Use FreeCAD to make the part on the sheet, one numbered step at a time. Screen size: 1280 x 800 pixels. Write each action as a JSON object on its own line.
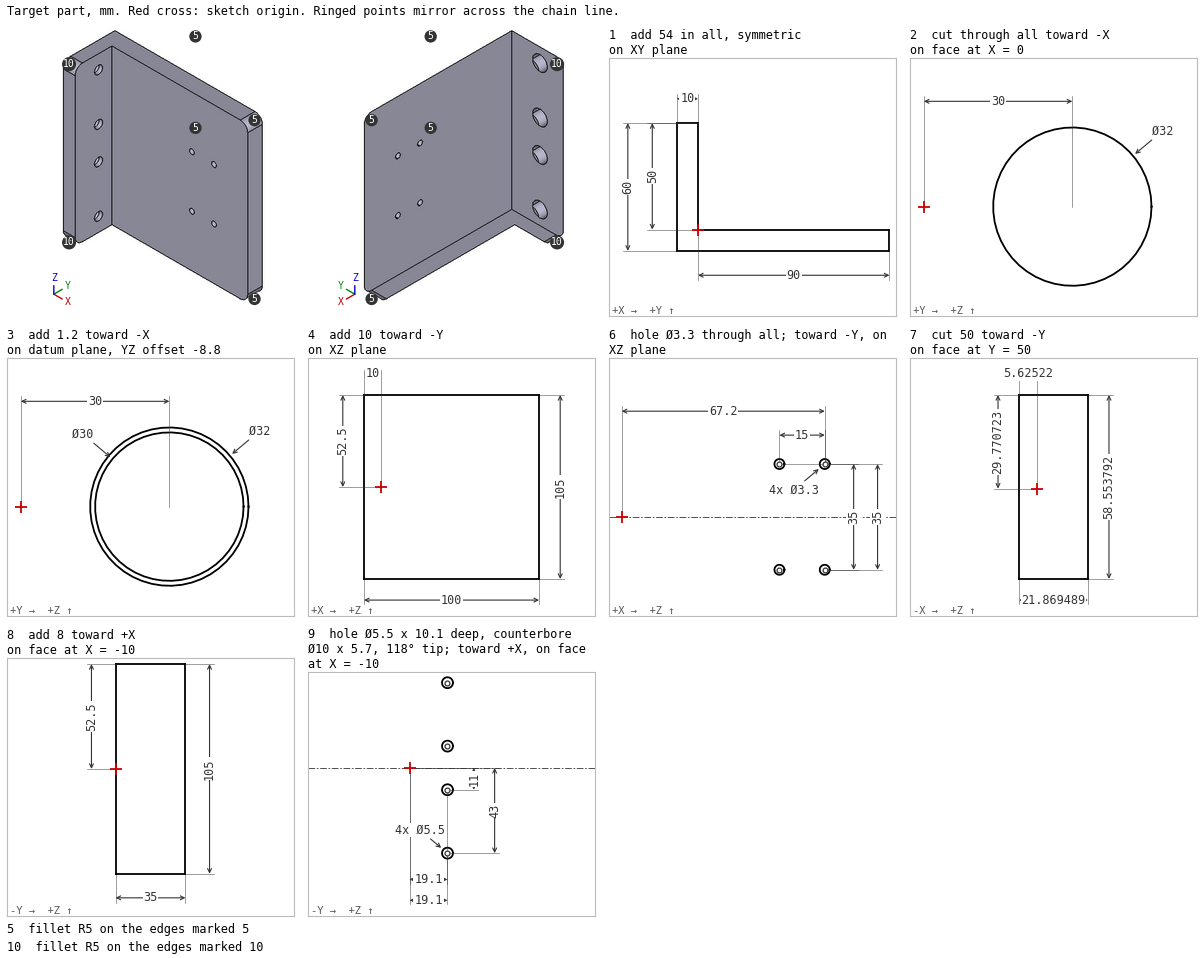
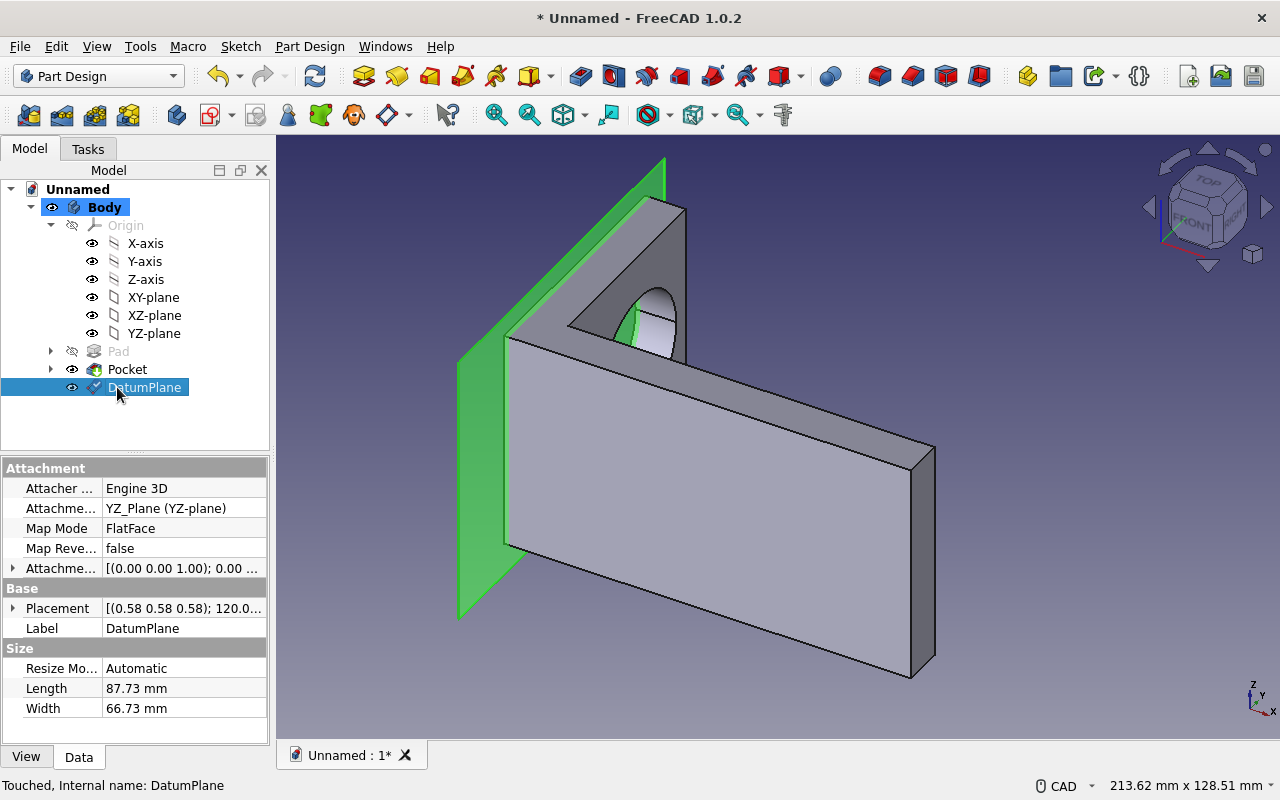
{"action": "left_click", "coordinate": [210, 116]}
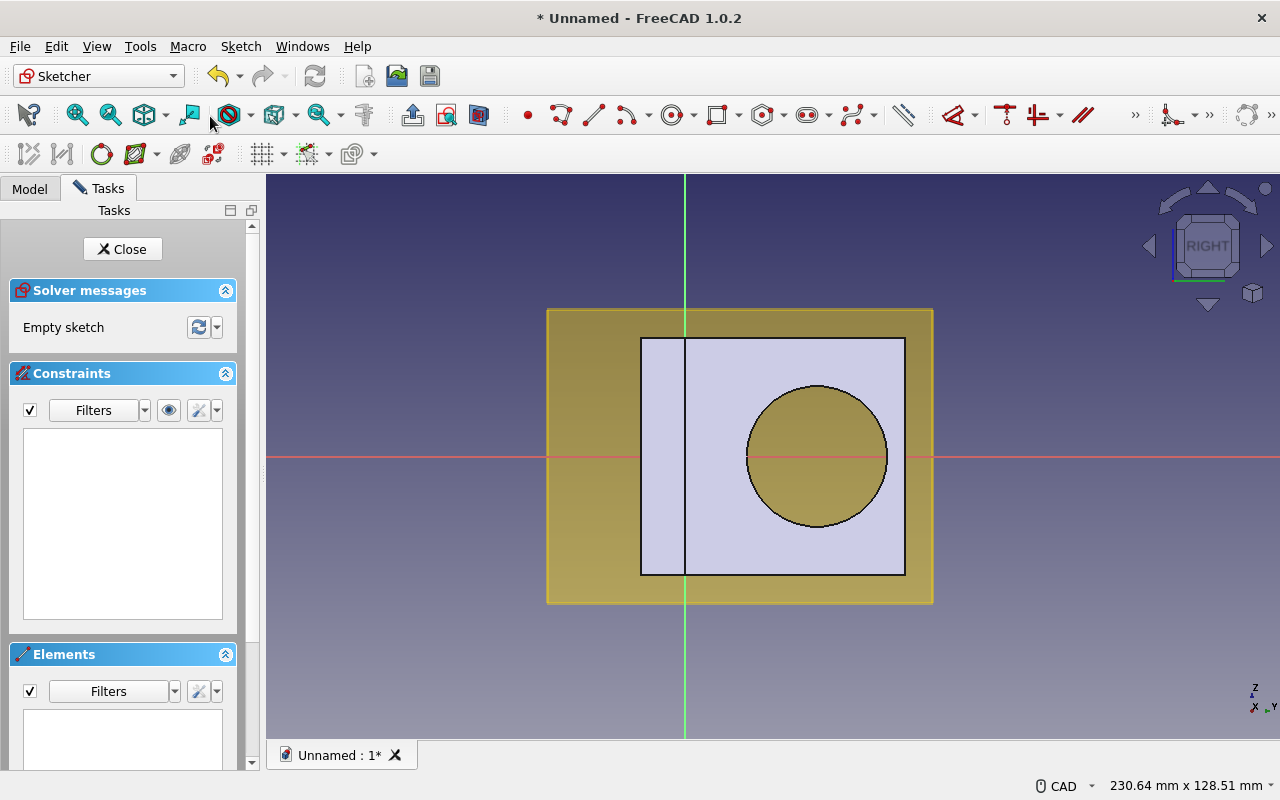
{"action": "left_click", "coordinate": [479, 116]}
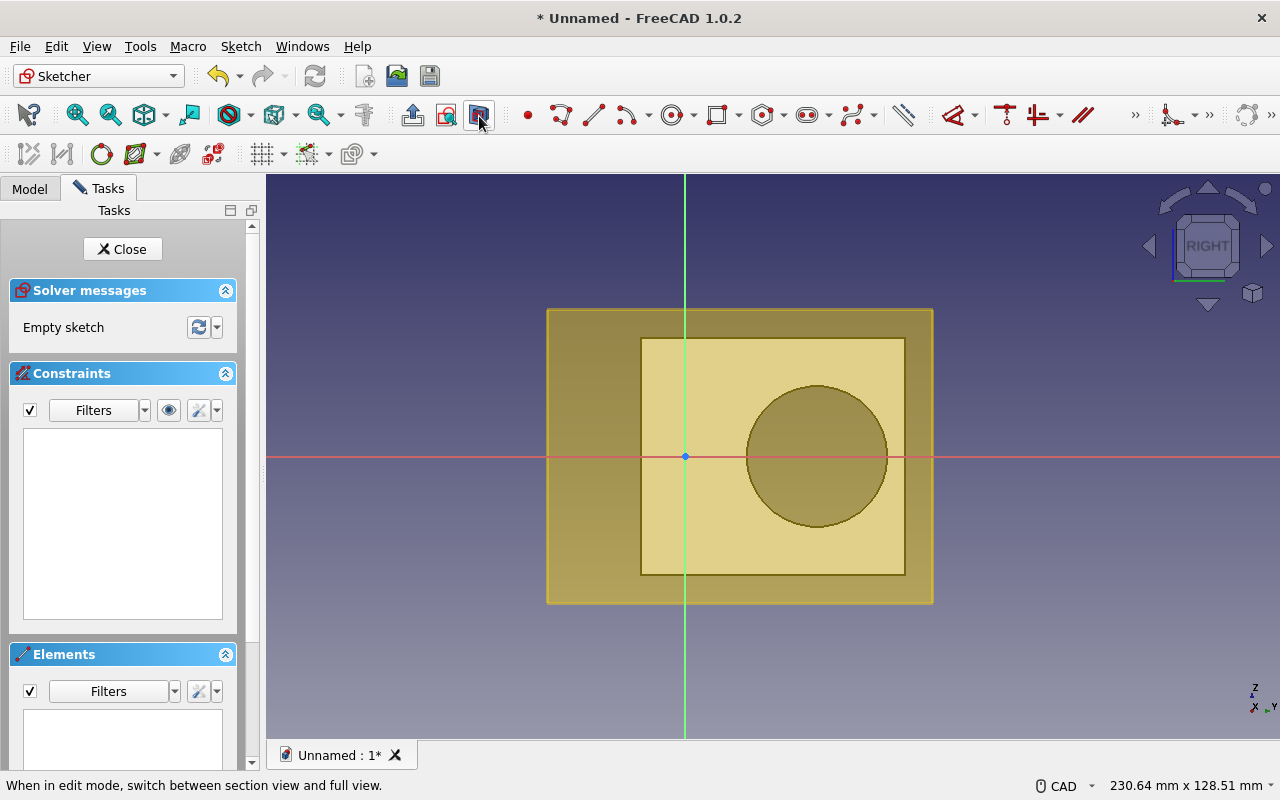
{"action": "scroll", "coordinate": [834, 456], "scroll_direction": "up", "scroll_amount": 5}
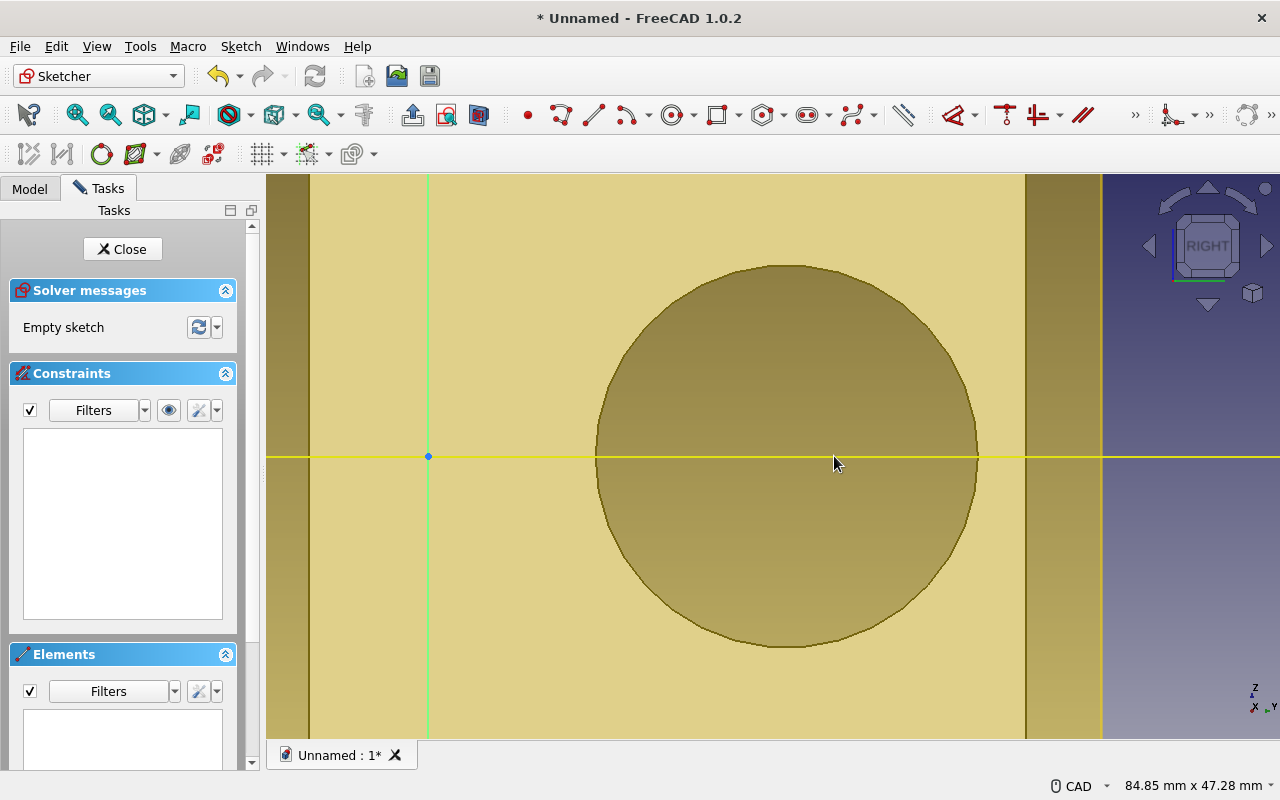
{"action": "left_click", "coordinate": [672, 116]}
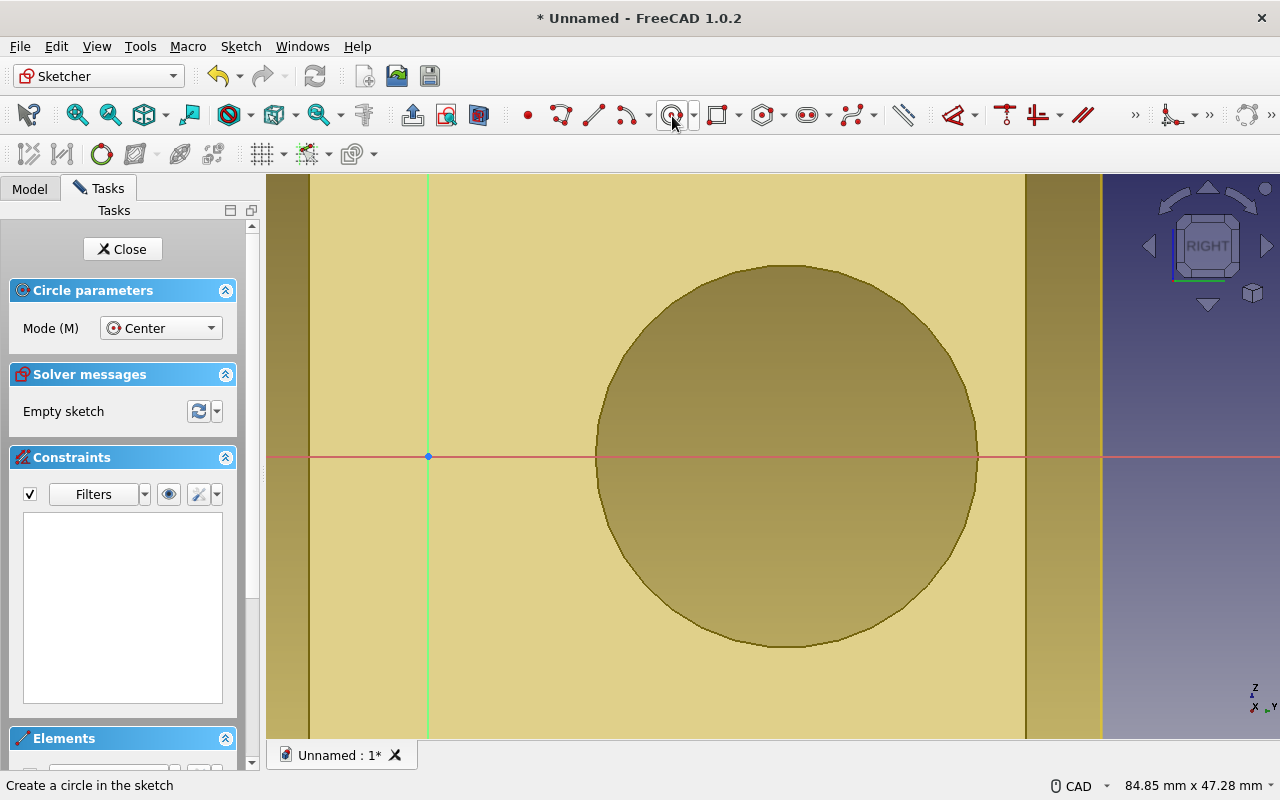
{"action": "left_click", "coordinate": [787, 456]}
{"action": "mouse_move", "coordinate": [922, 321]}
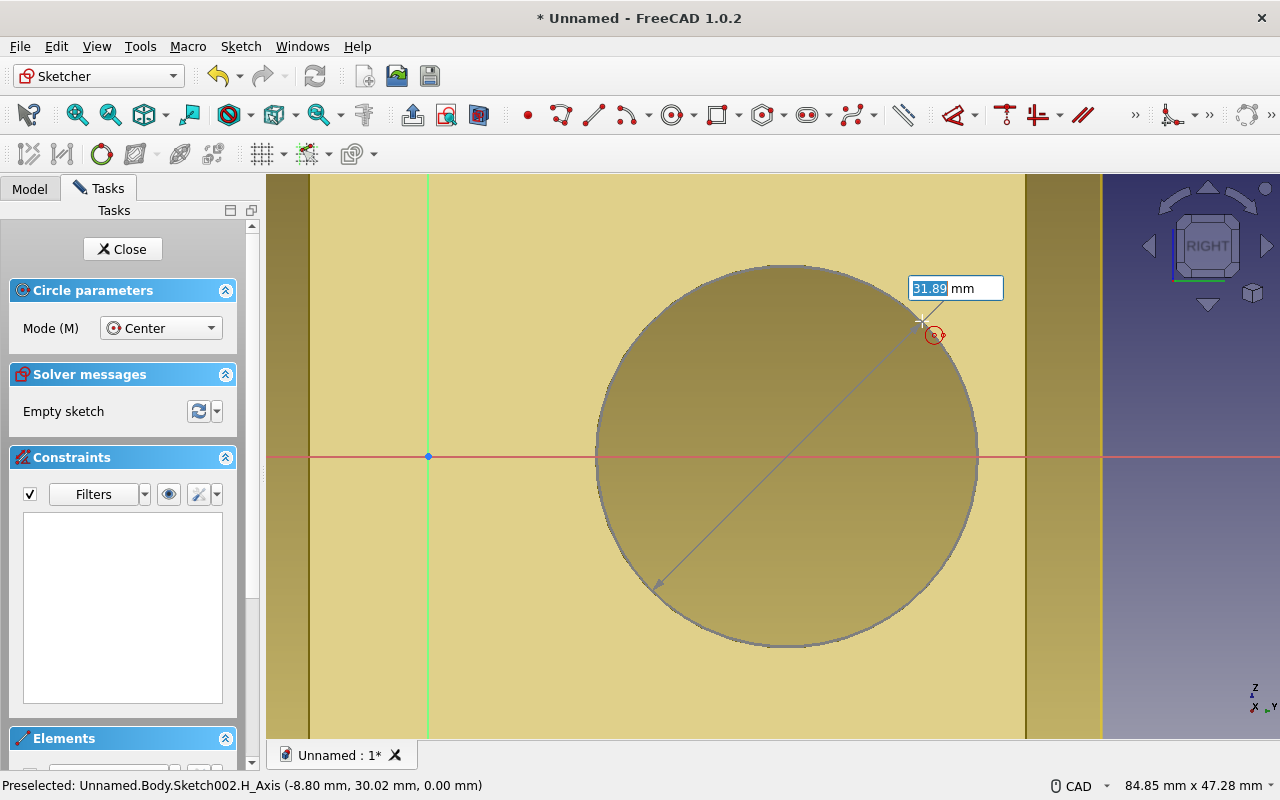
{"action": "type", "text": "32"}
{"action": "key", "text": "Return"}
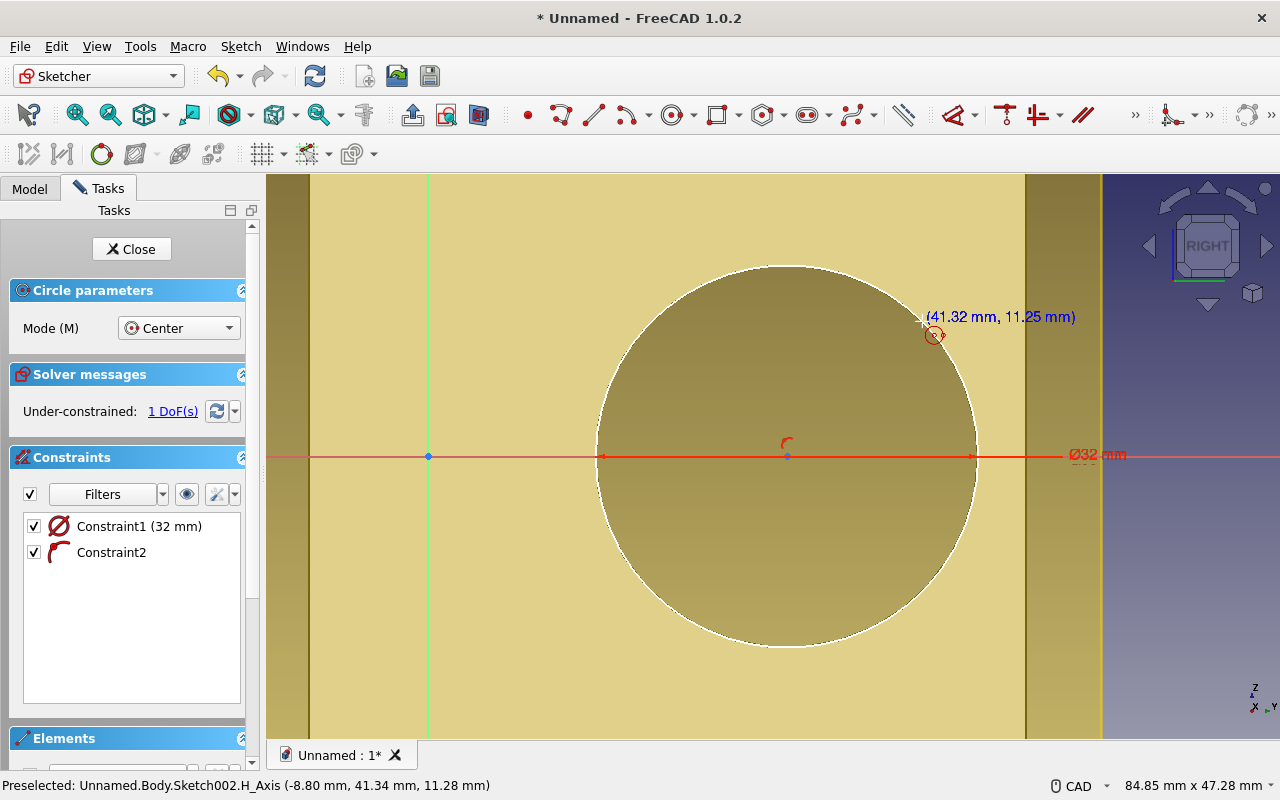
{"action": "left_click", "coordinate": [787, 456]}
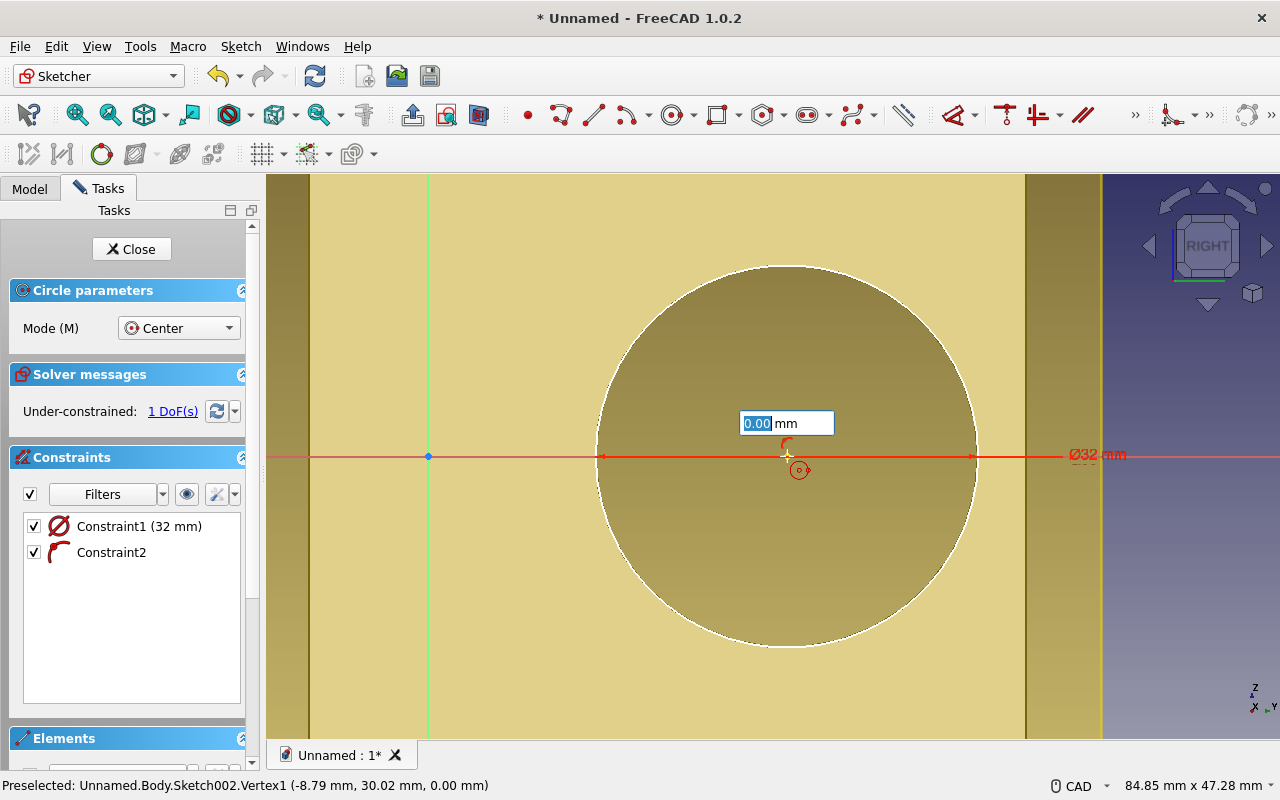
{"action": "scroll", "coordinate": [955, 395], "scroll_direction": "up", "scroll_amount": 2}
{"action": "mouse_move", "coordinate": [955, 395]}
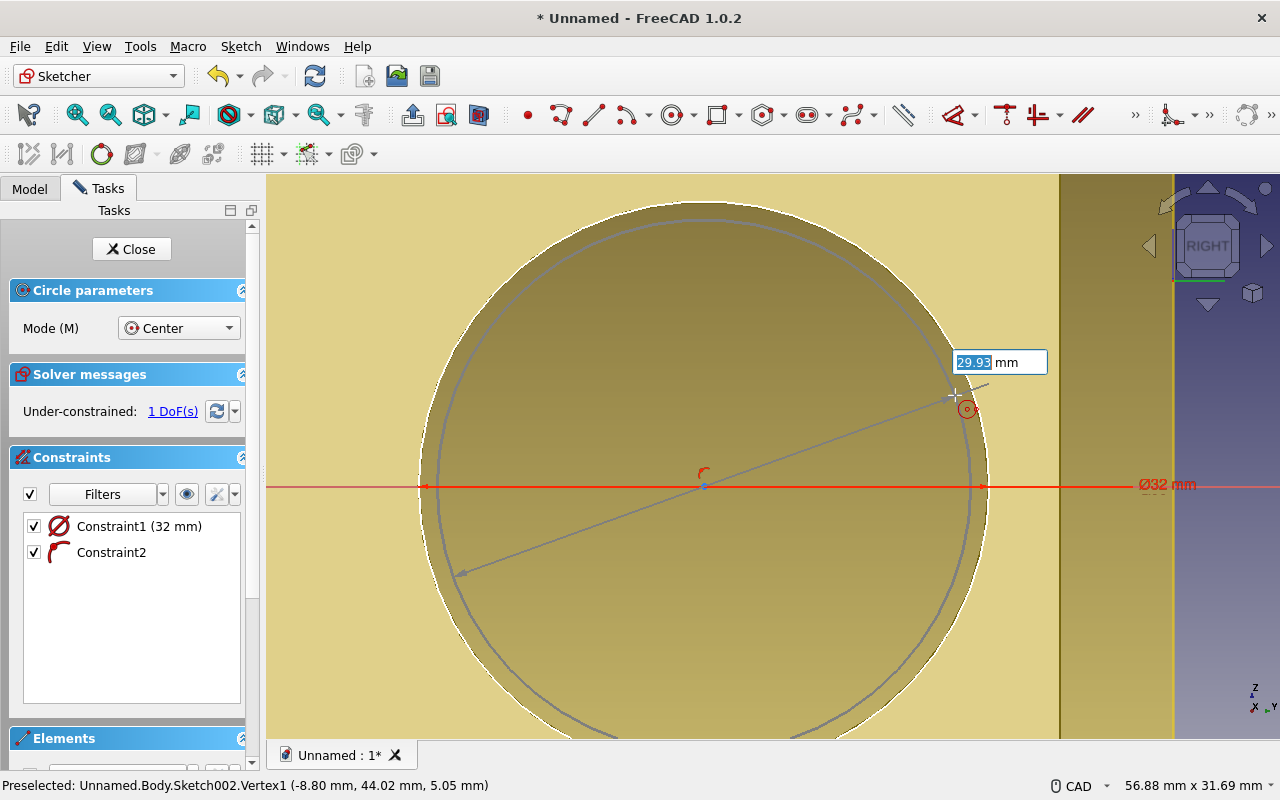
{"action": "type", "text": "30"}
{"action": "key", "text": "Return"}
{"action": "key", "text": "Escape"}